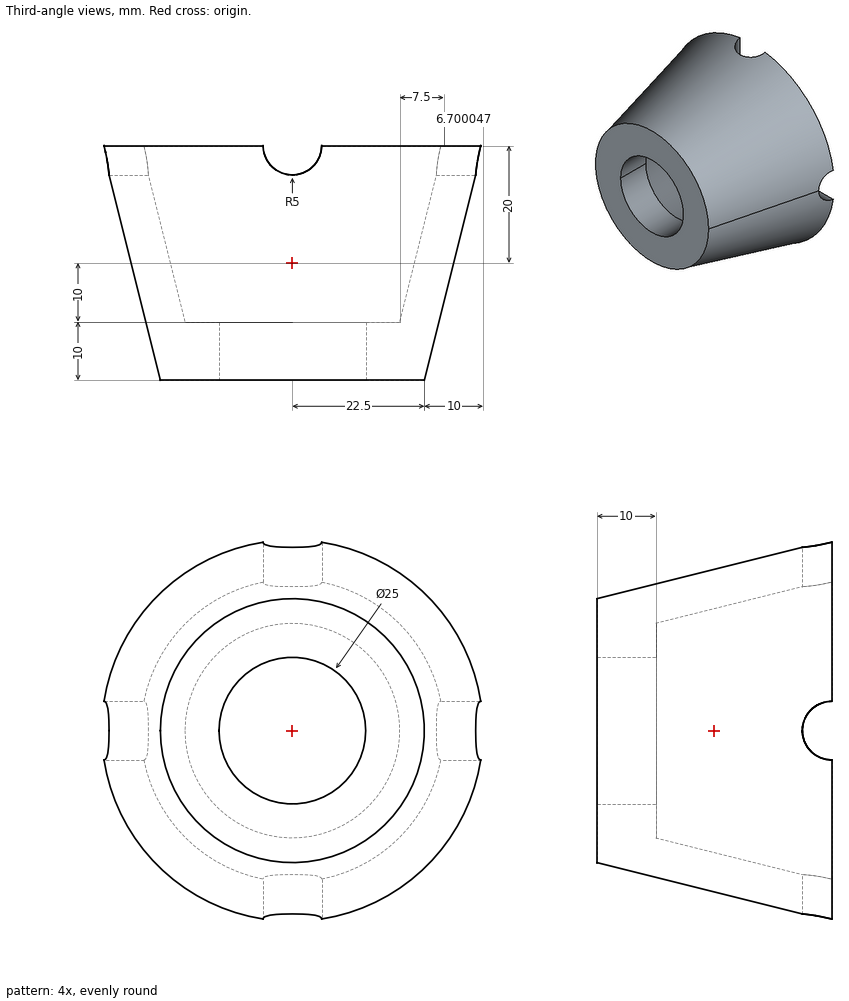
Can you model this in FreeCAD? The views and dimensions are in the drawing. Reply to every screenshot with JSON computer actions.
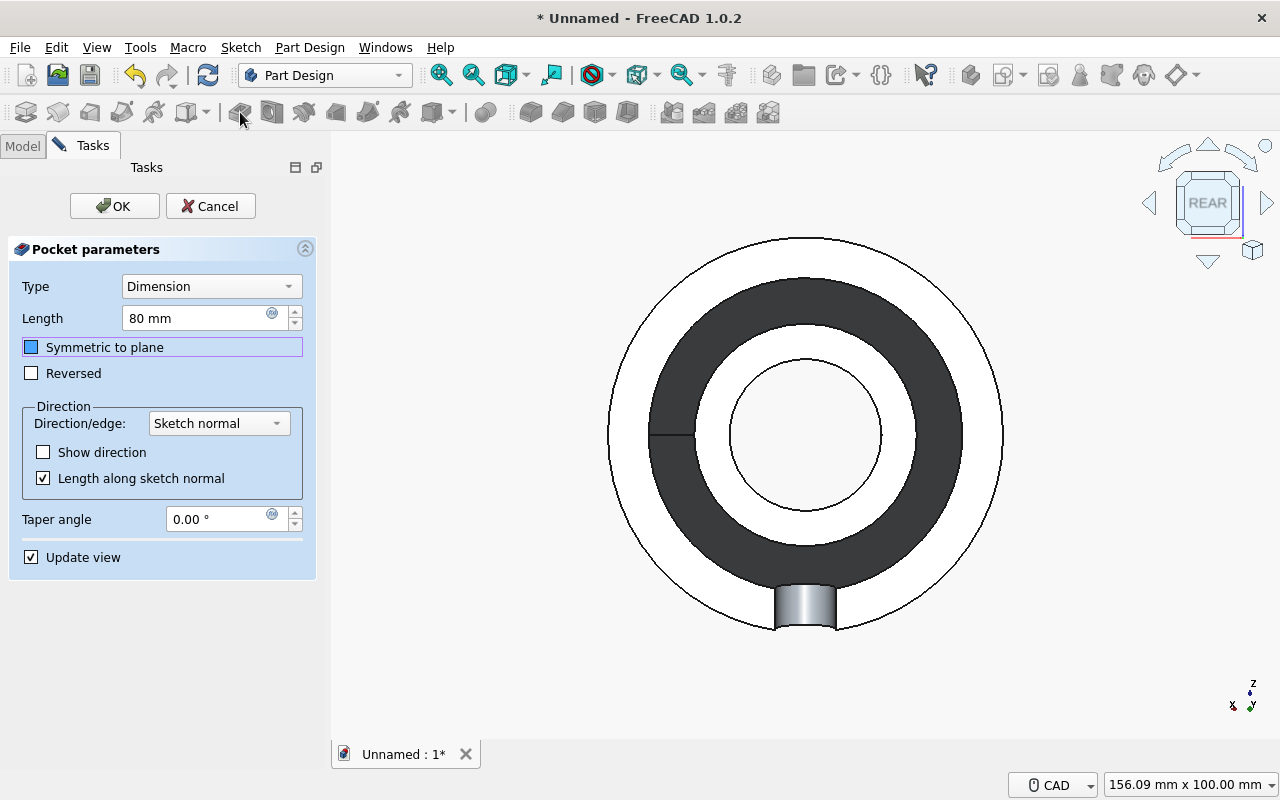
{"action": "left_click", "coordinate": [30, 347]}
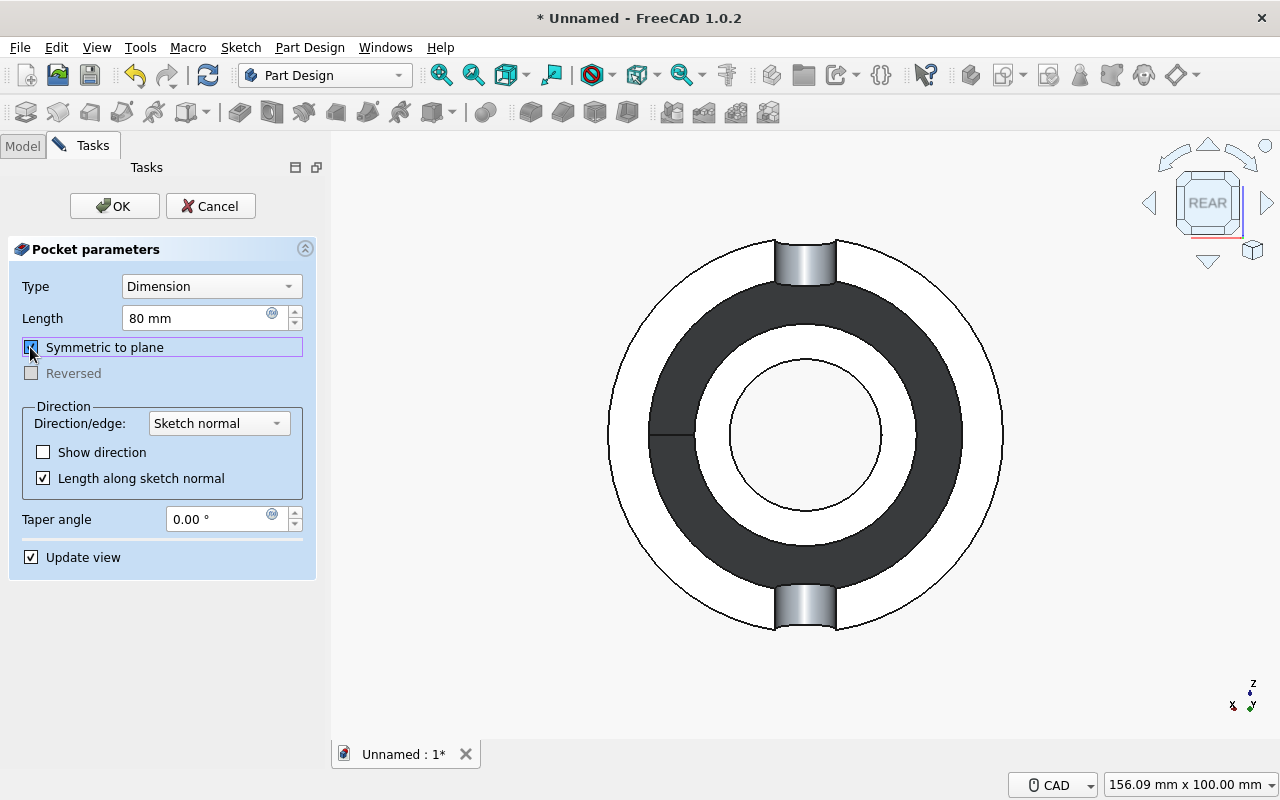
{"action": "left_click", "coordinate": [115, 206]}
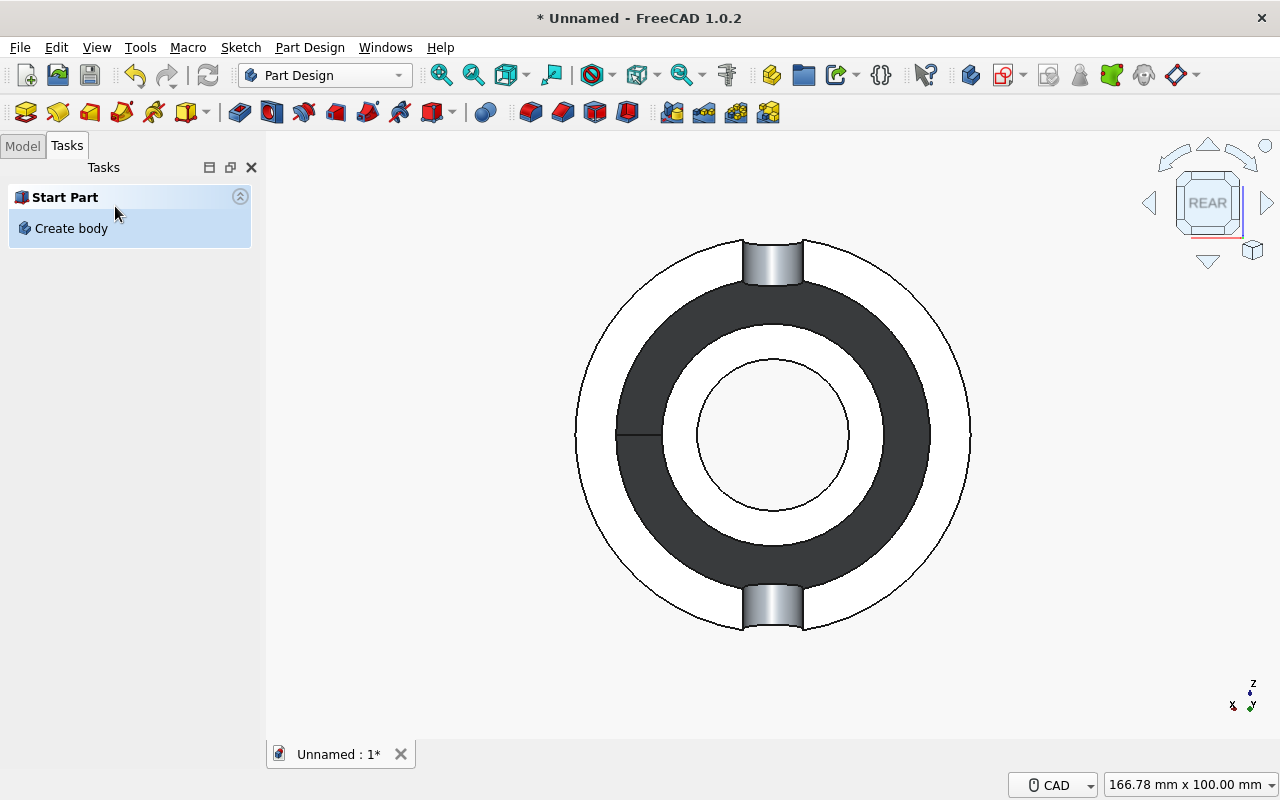
{"action": "left_click", "coordinate": [23, 145]}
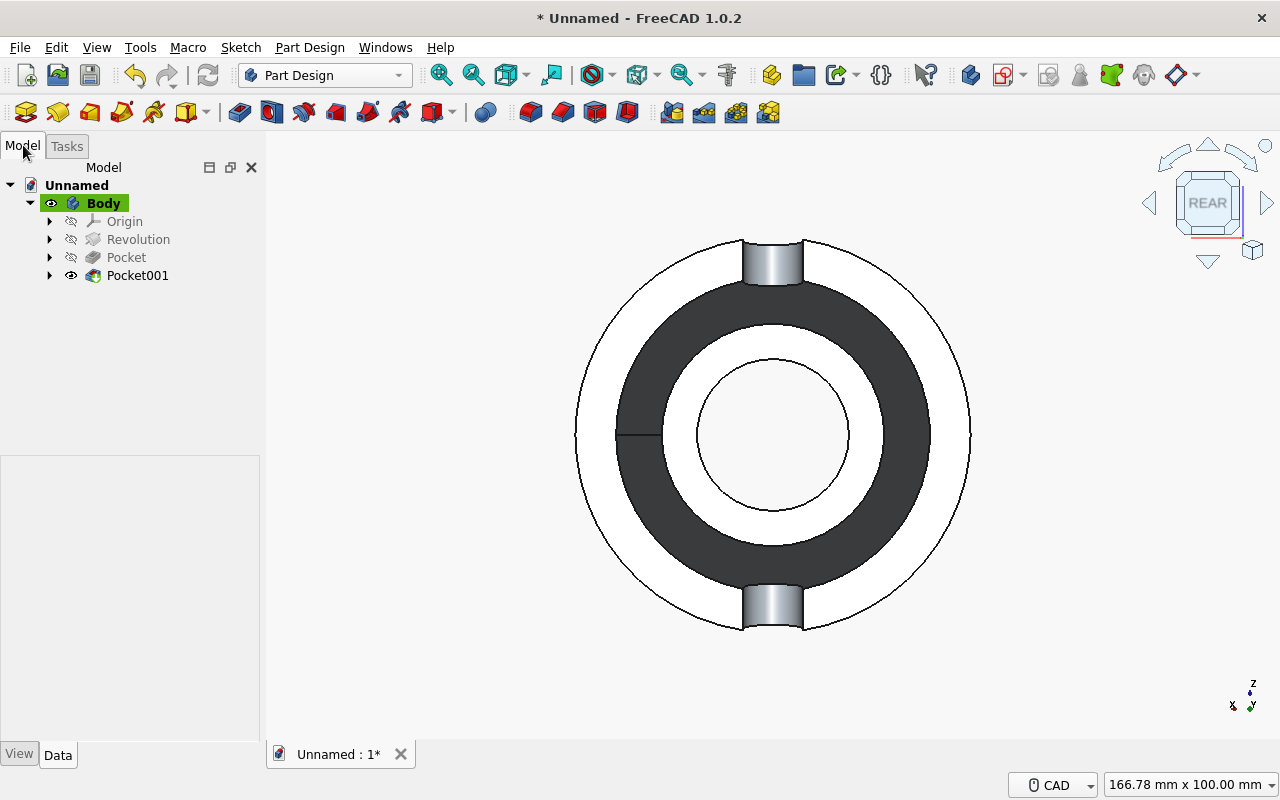
{"action": "left_click", "coordinate": [116, 275]}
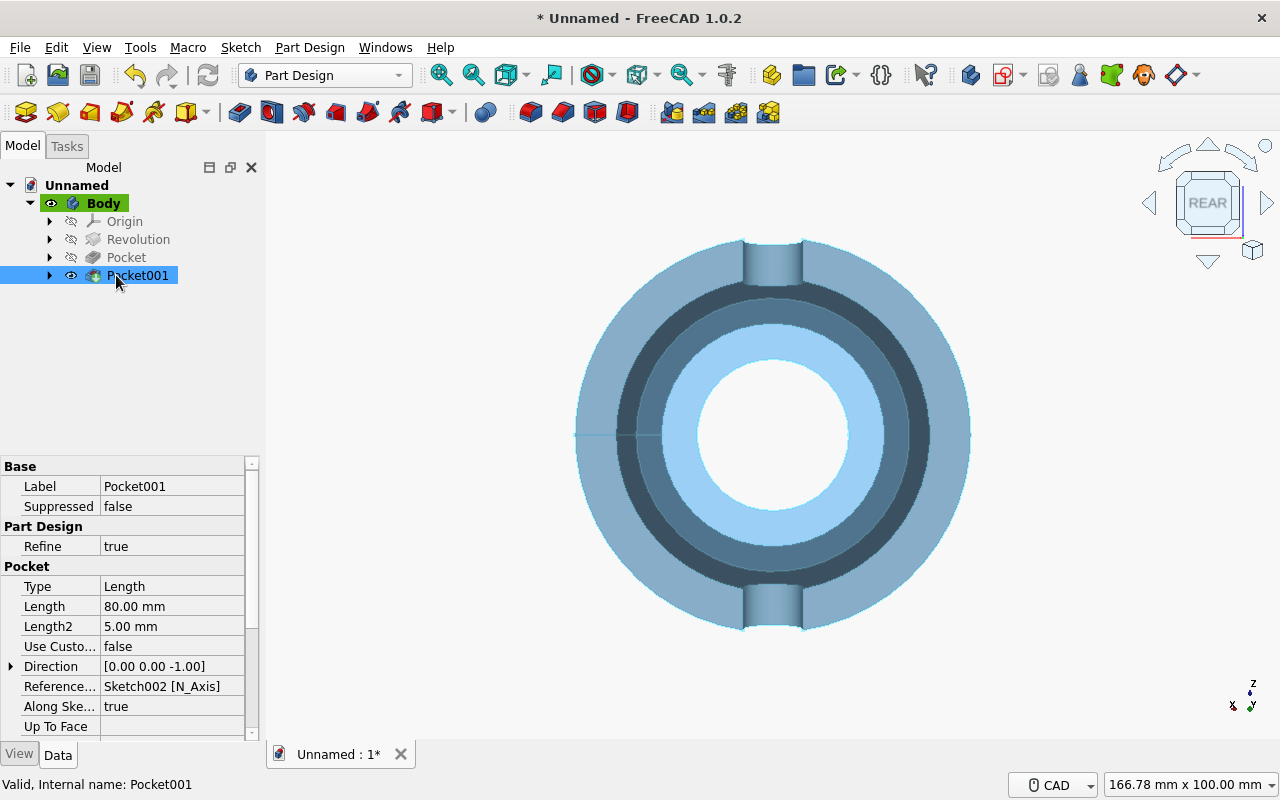
{"action": "left_click", "coordinate": [736, 112]}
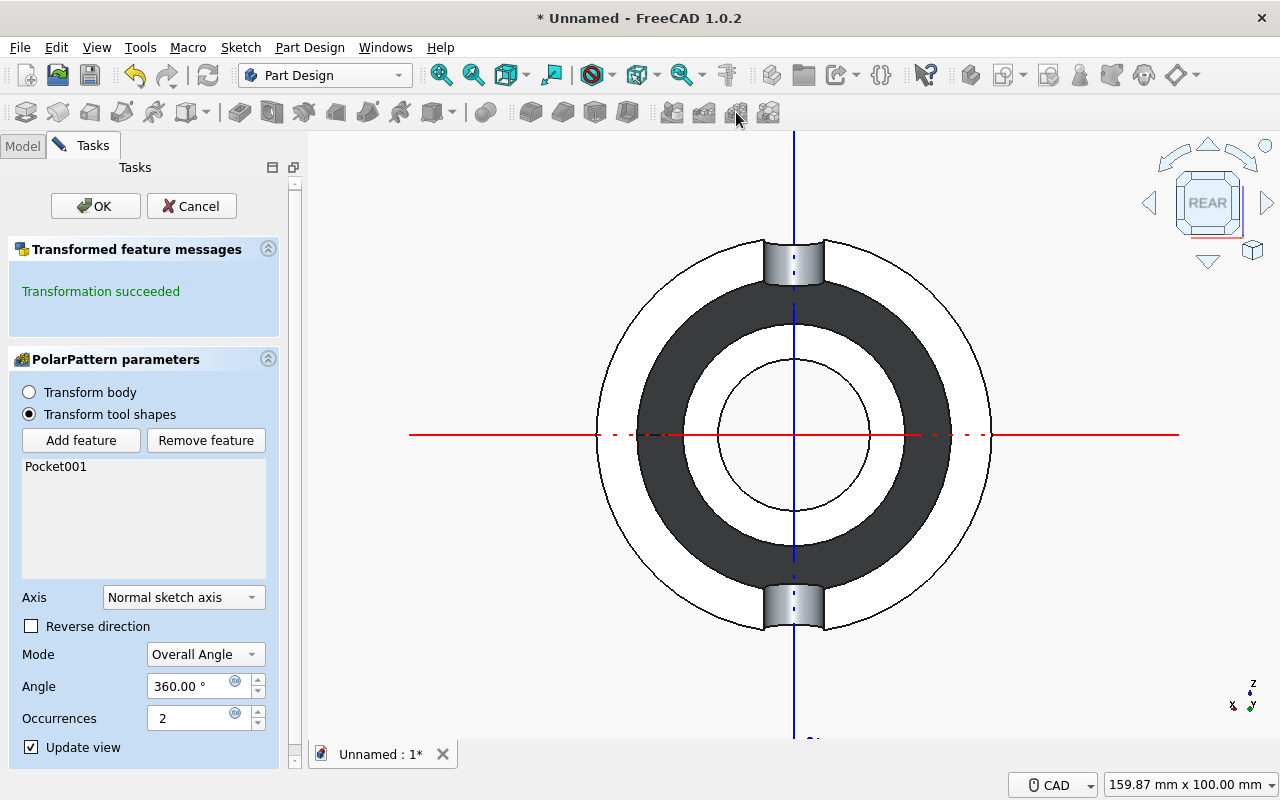
{"action": "left_click", "coordinate": [184, 598]}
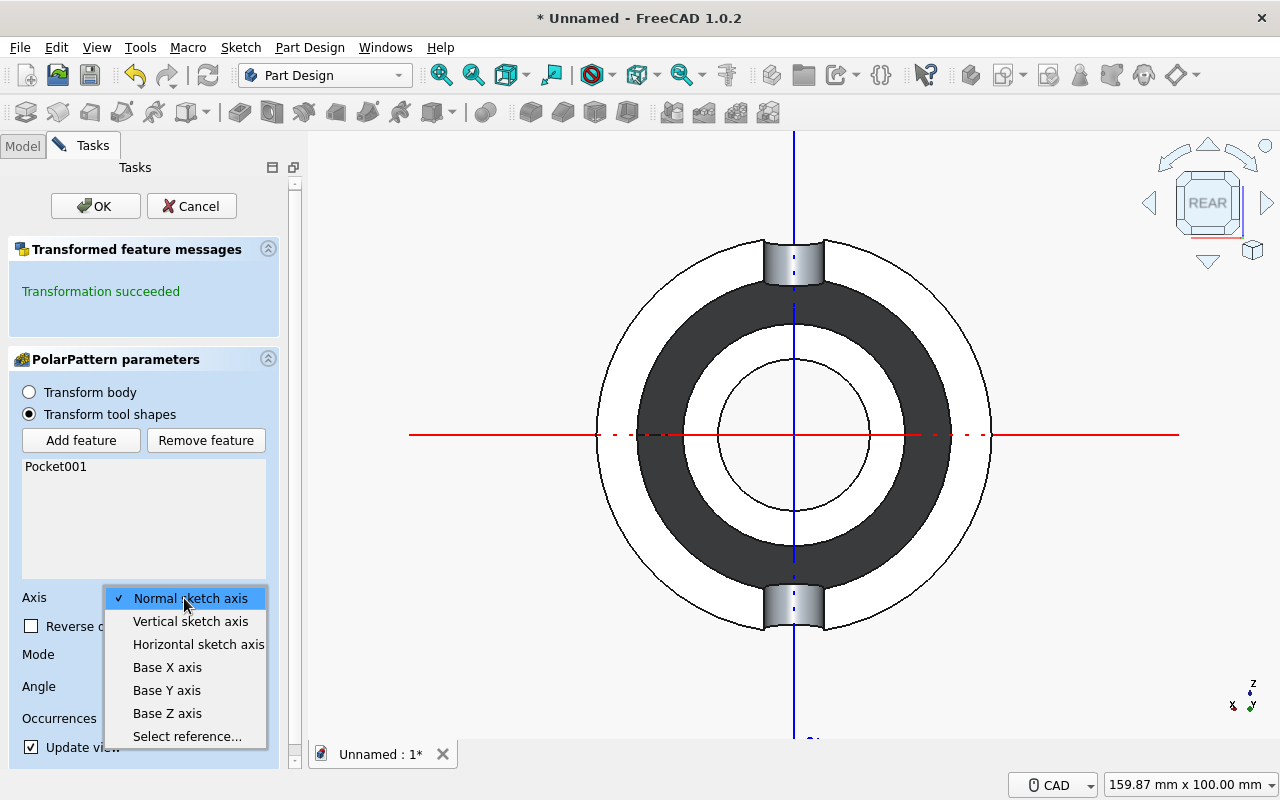
{"action": "left_click", "coordinate": [184, 690]}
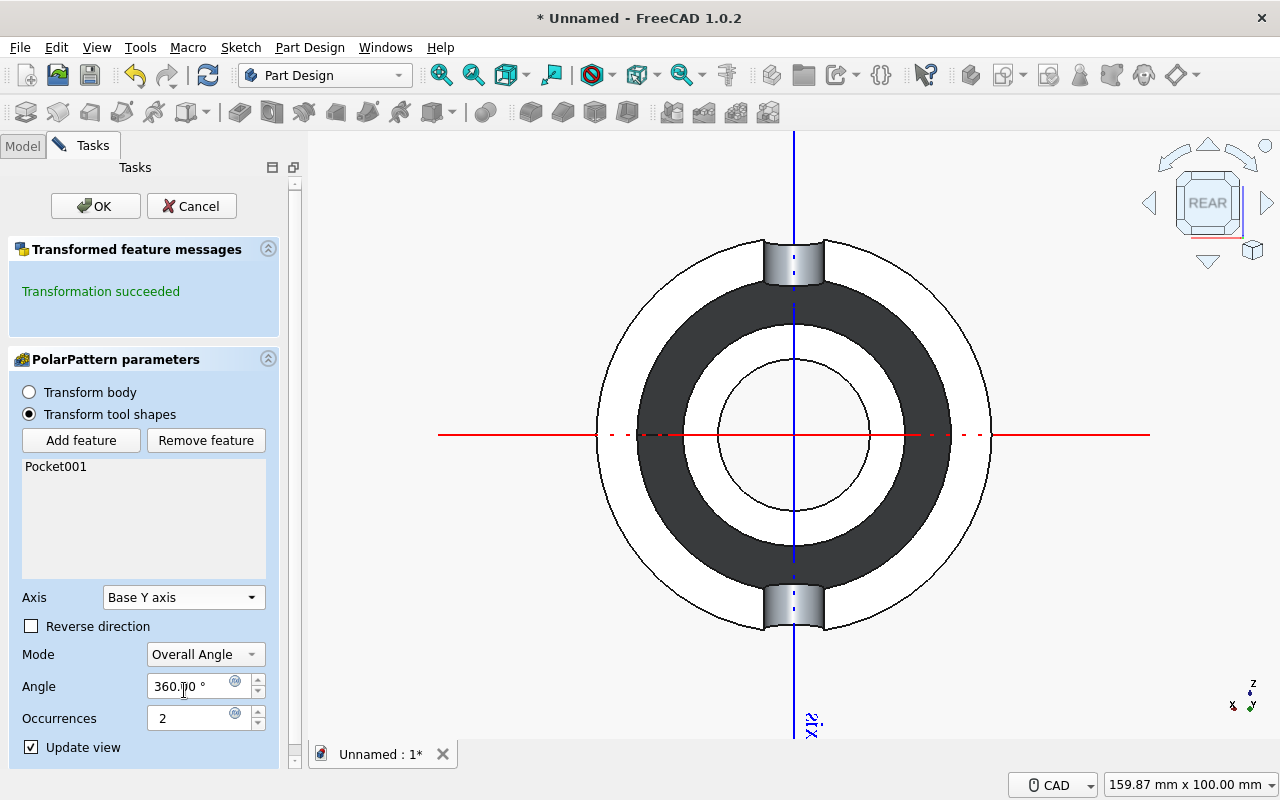
{"action": "triple_click", "coordinate": [198, 718]}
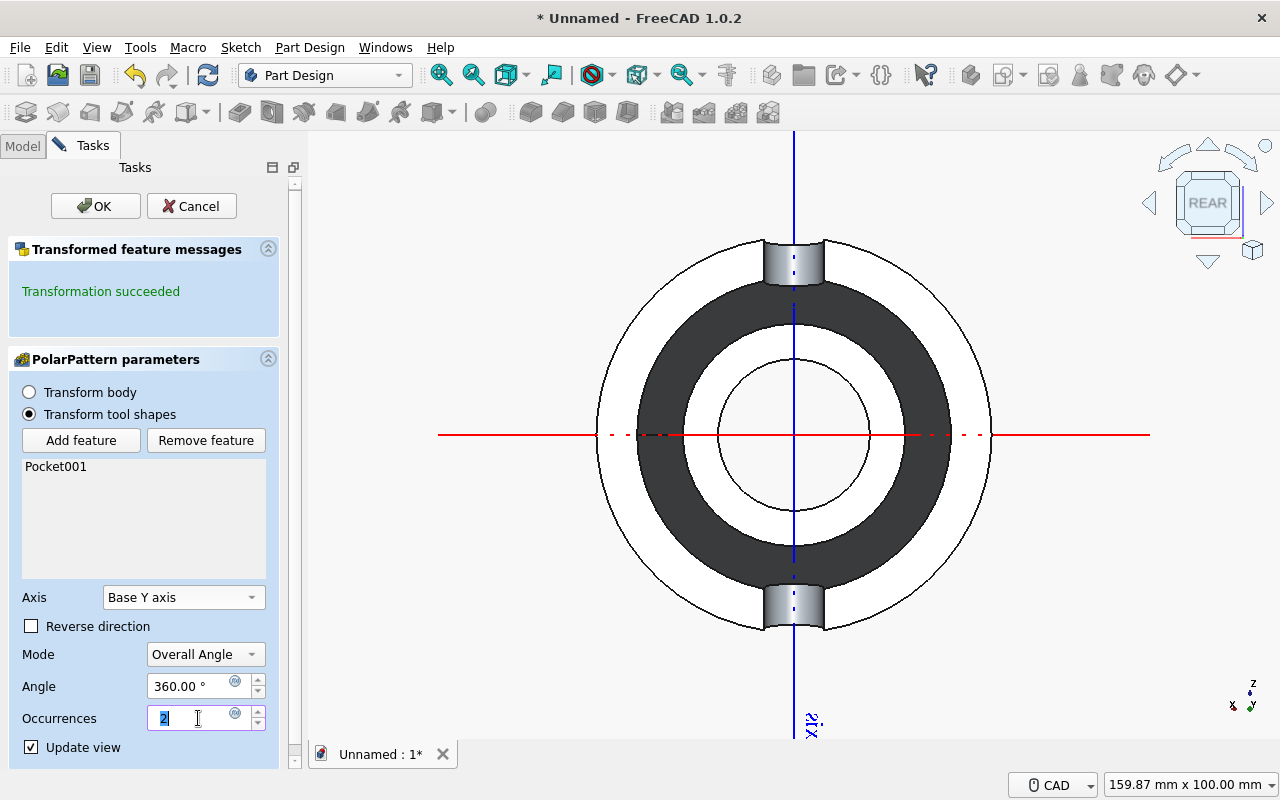
{"action": "type", "text": "4"}
{"action": "key", "text": "Tab"}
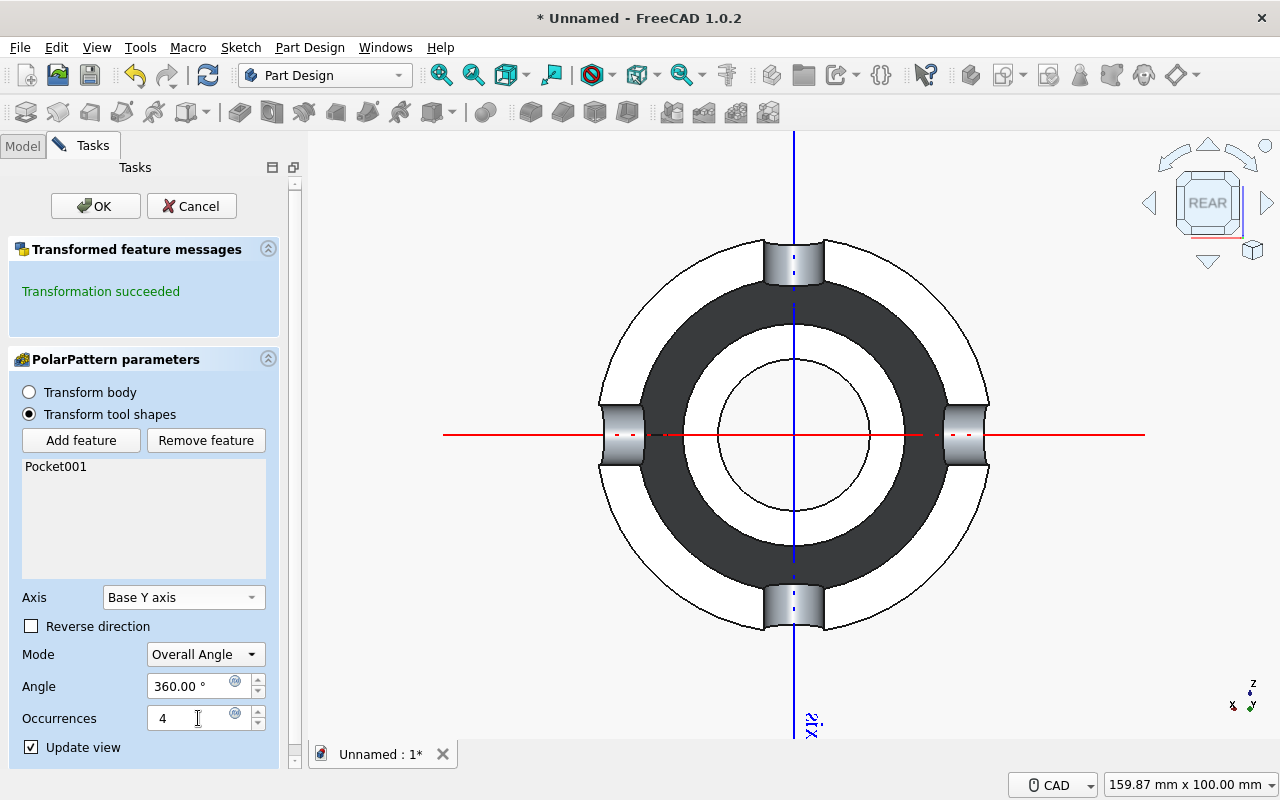
{"action": "left_click", "coordinate": [96, 206]}